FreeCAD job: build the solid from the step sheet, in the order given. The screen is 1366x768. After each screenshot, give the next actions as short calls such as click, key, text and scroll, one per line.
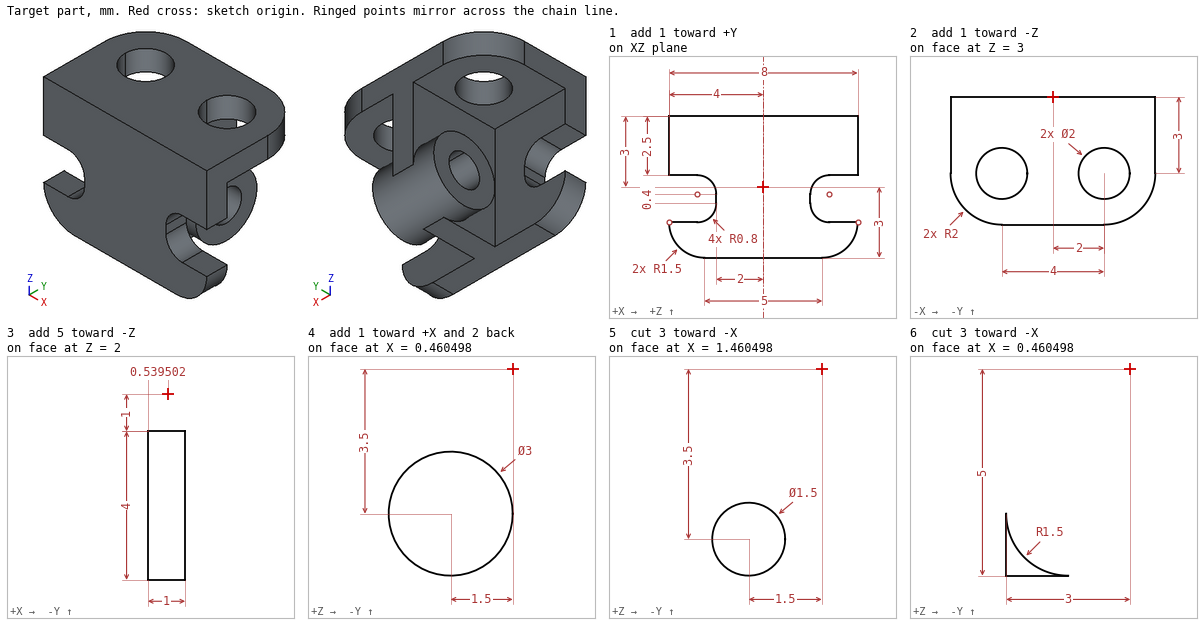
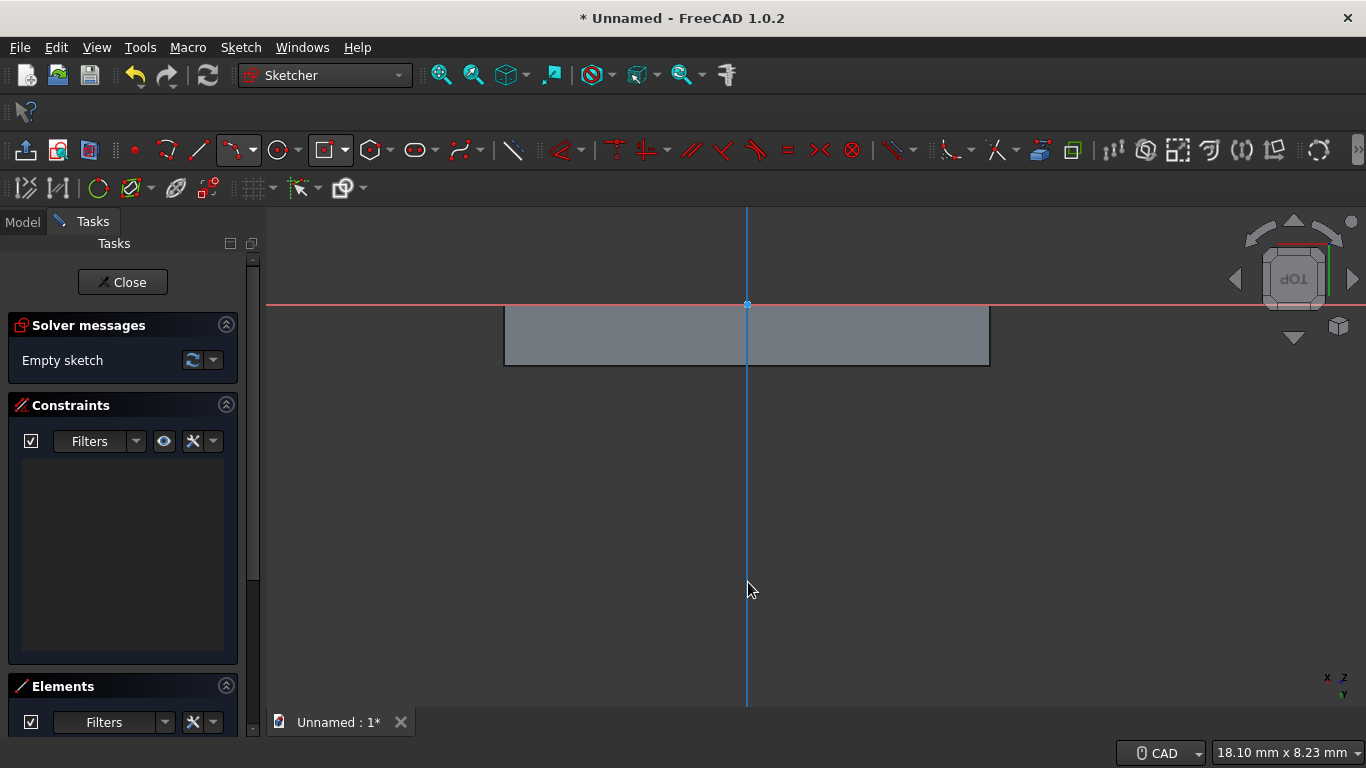
click(200, 150)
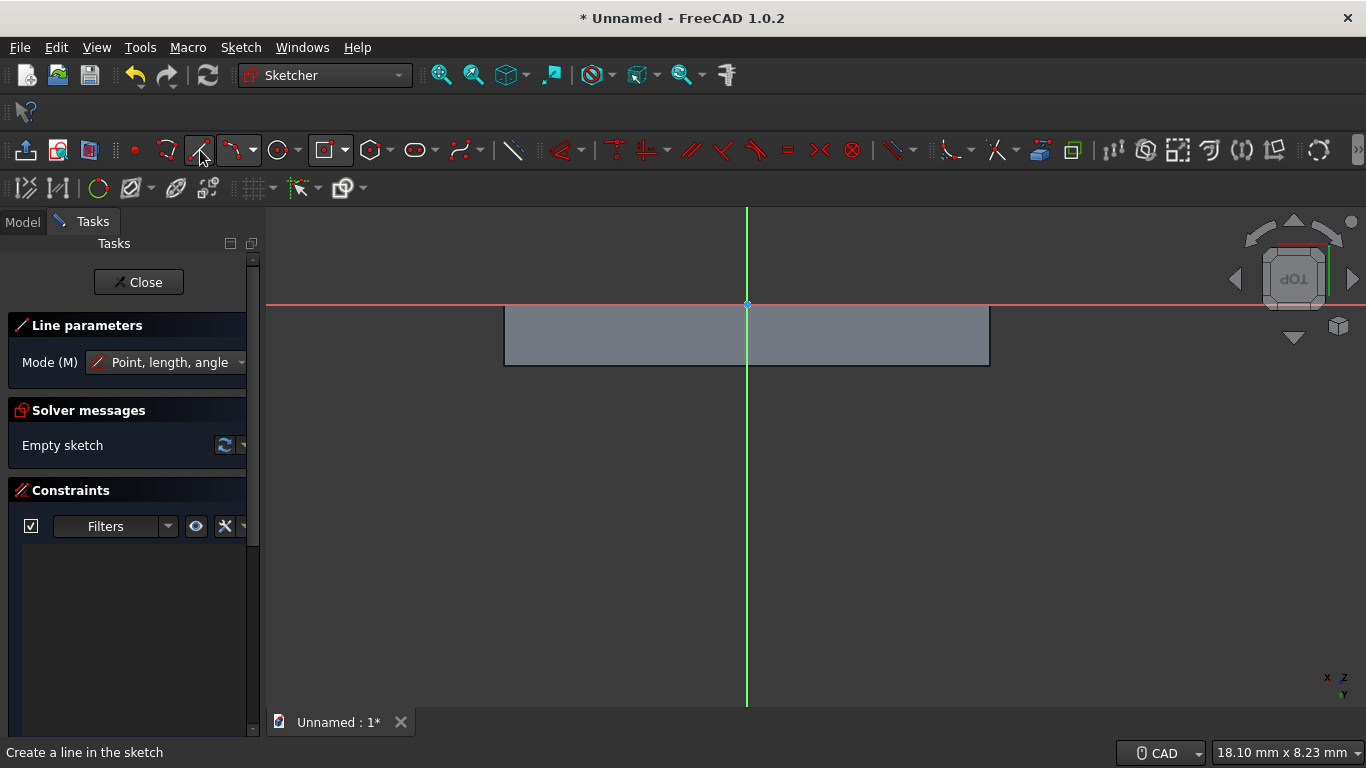
click(626, 609)
click(869, 609)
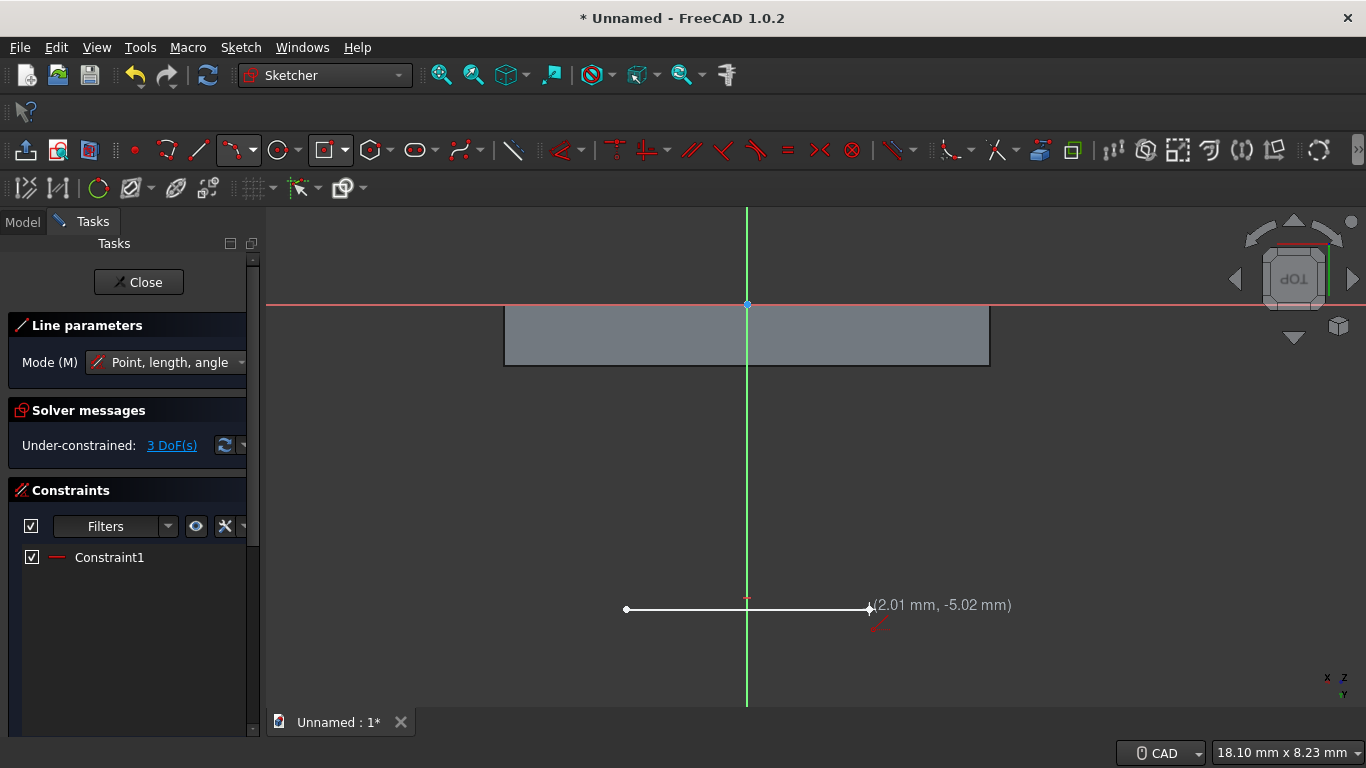
click(168, 150)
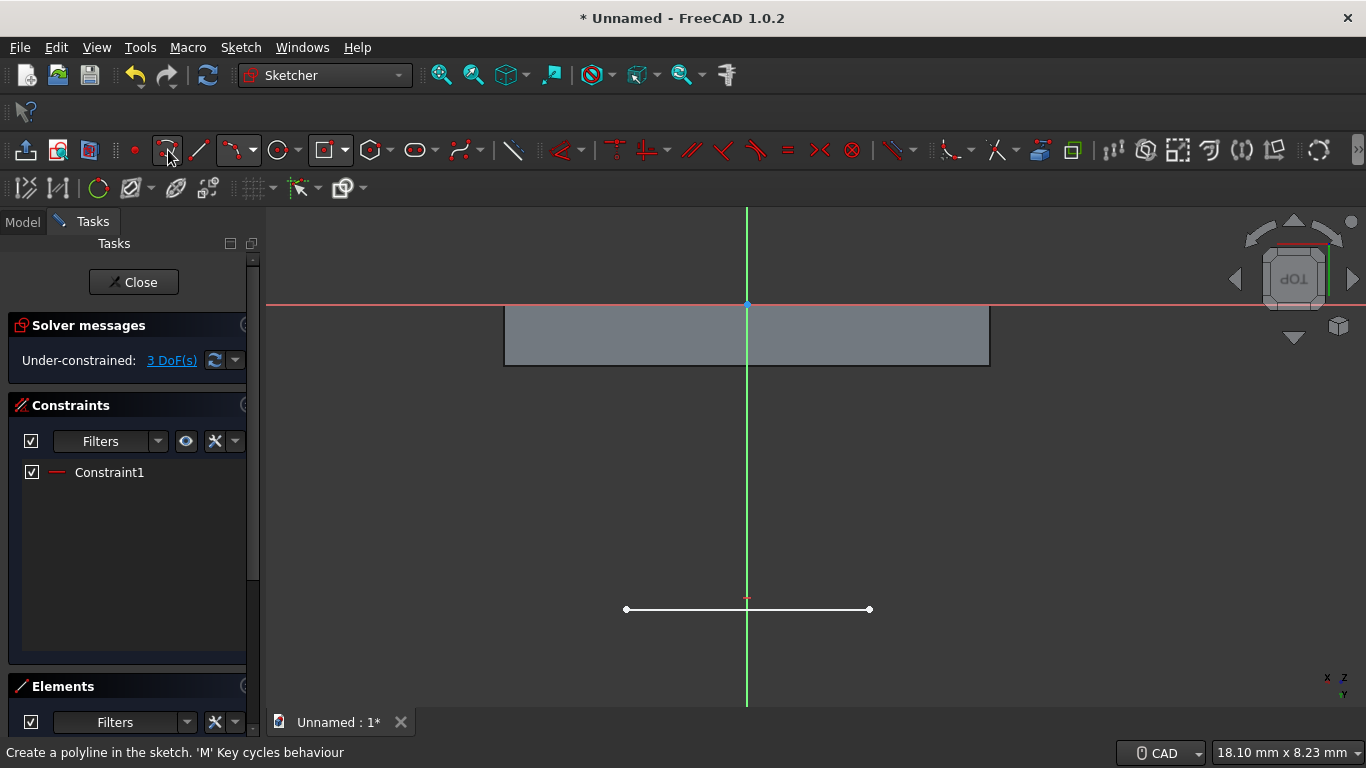
click(990, 487)
click(990, 305)
click(504, 314)
click(504, 487)
right_click(504, 487)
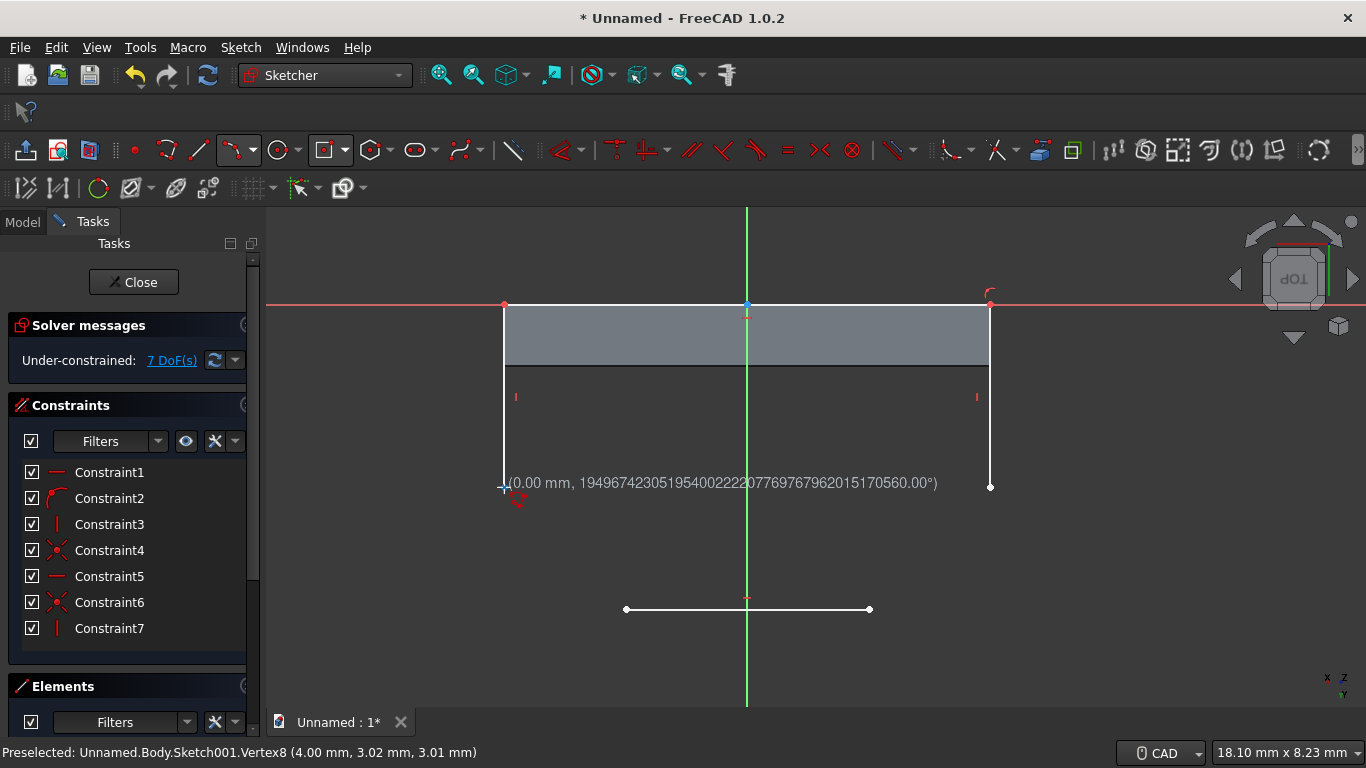
click(232, 150)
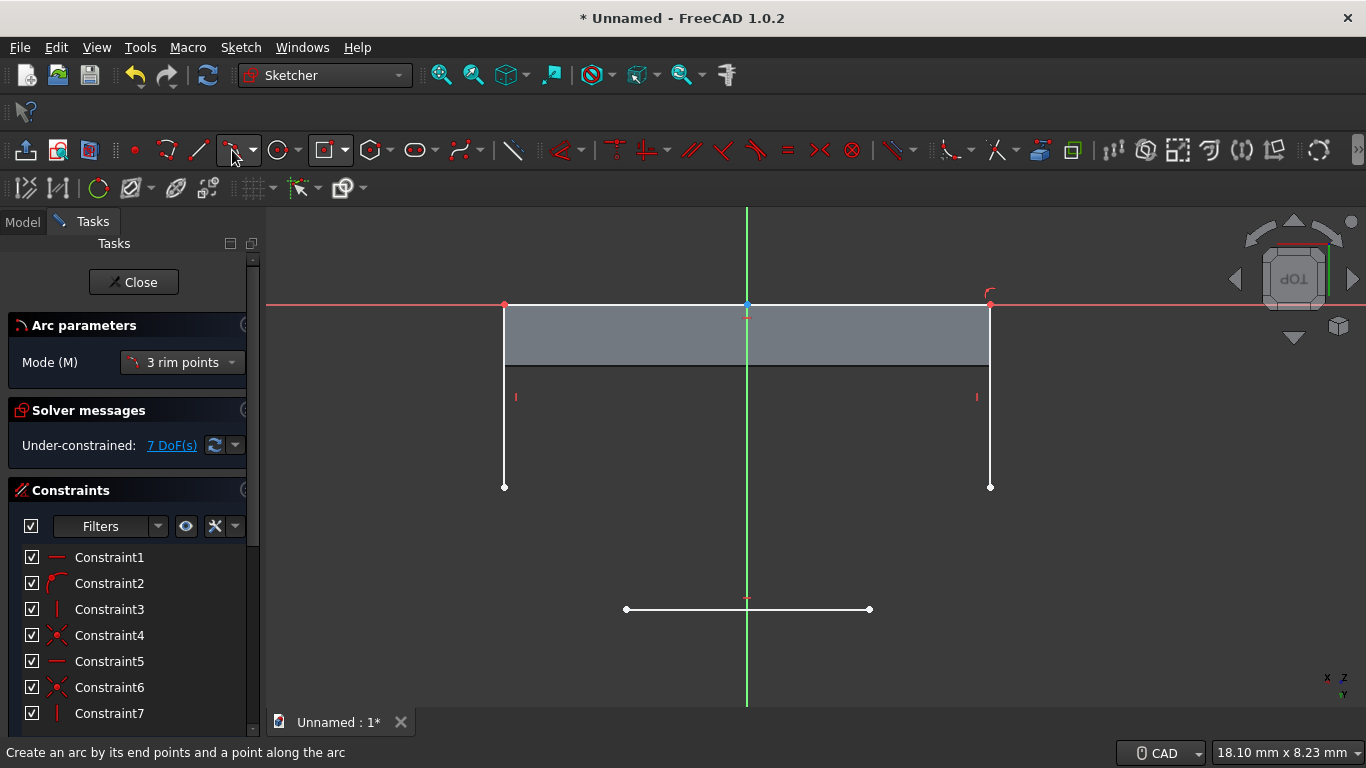
click(869, 610)
click(990, 488)
click(955, 573)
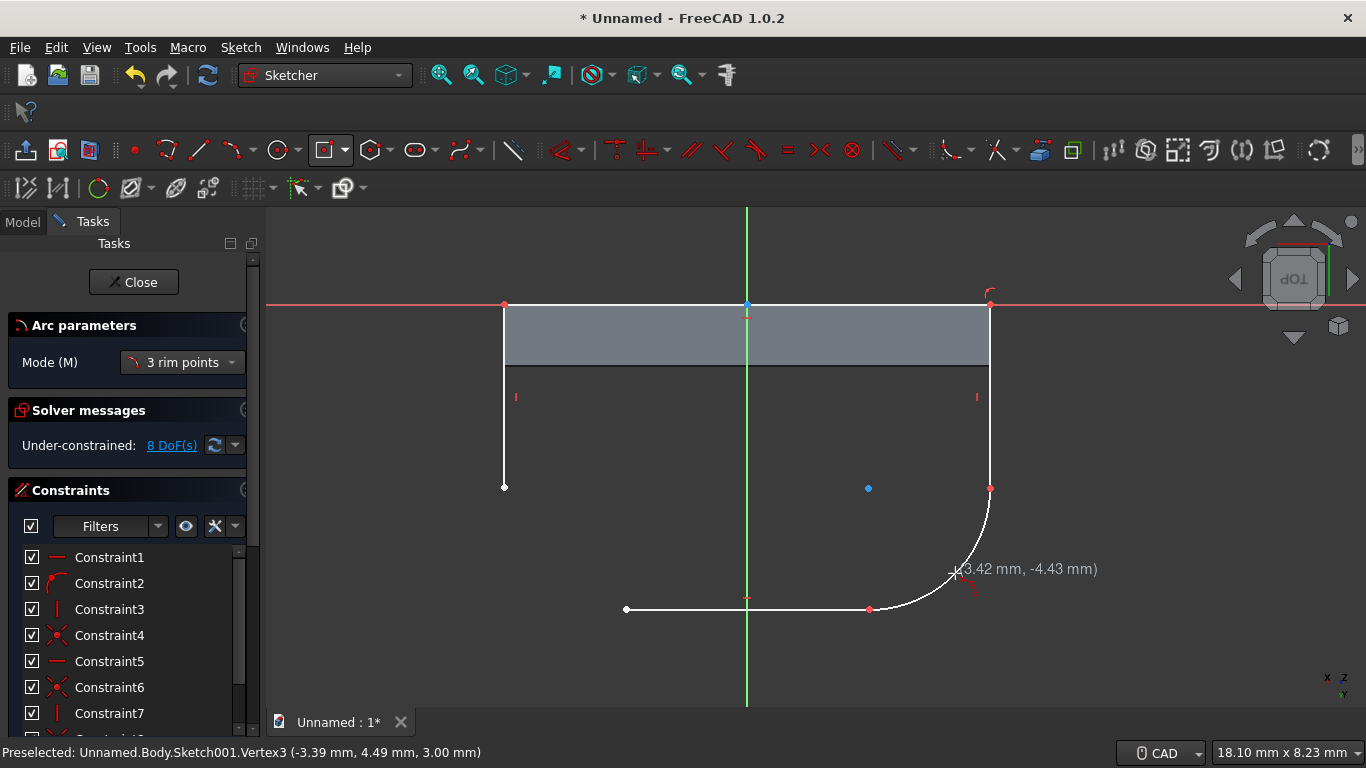
click(504, 488)
click(626, 610)
click(540, 573)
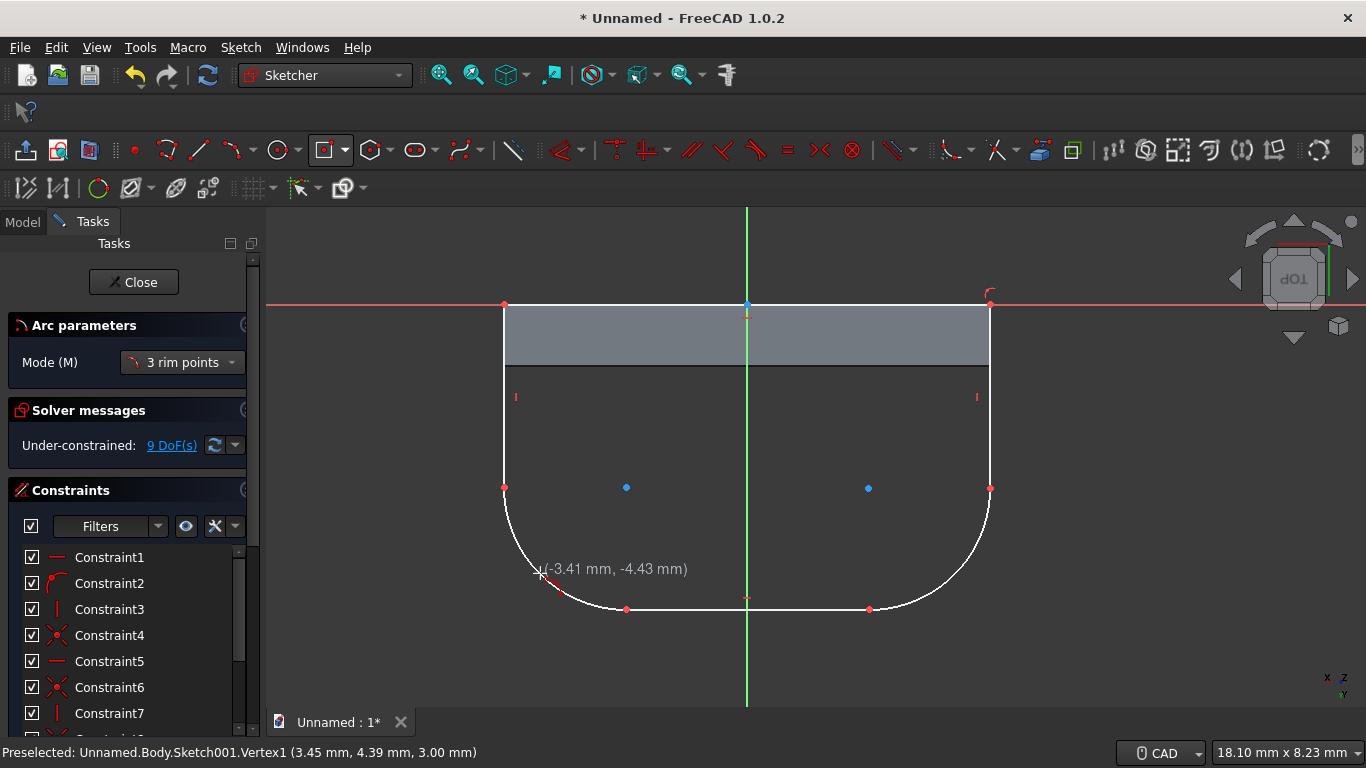
click(278, 150)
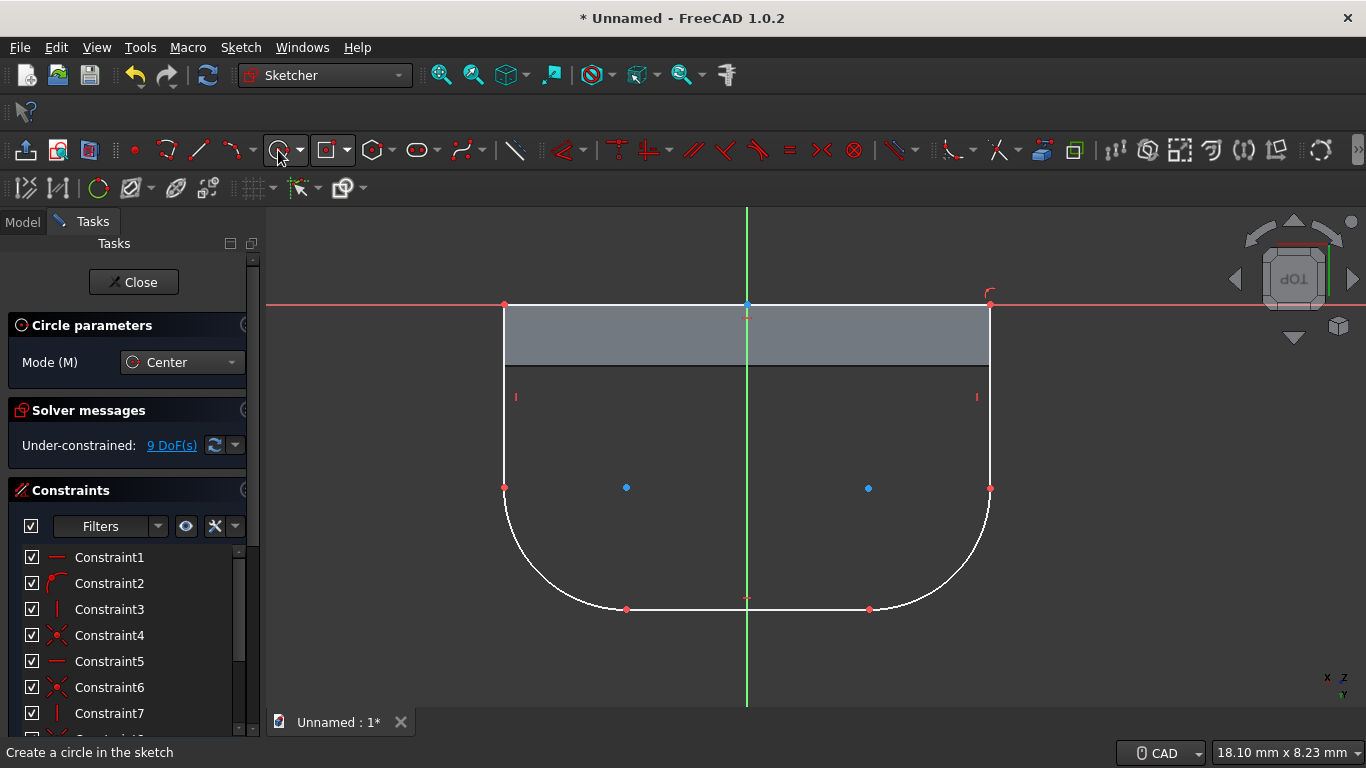
click(869, 487)
click(912, 444)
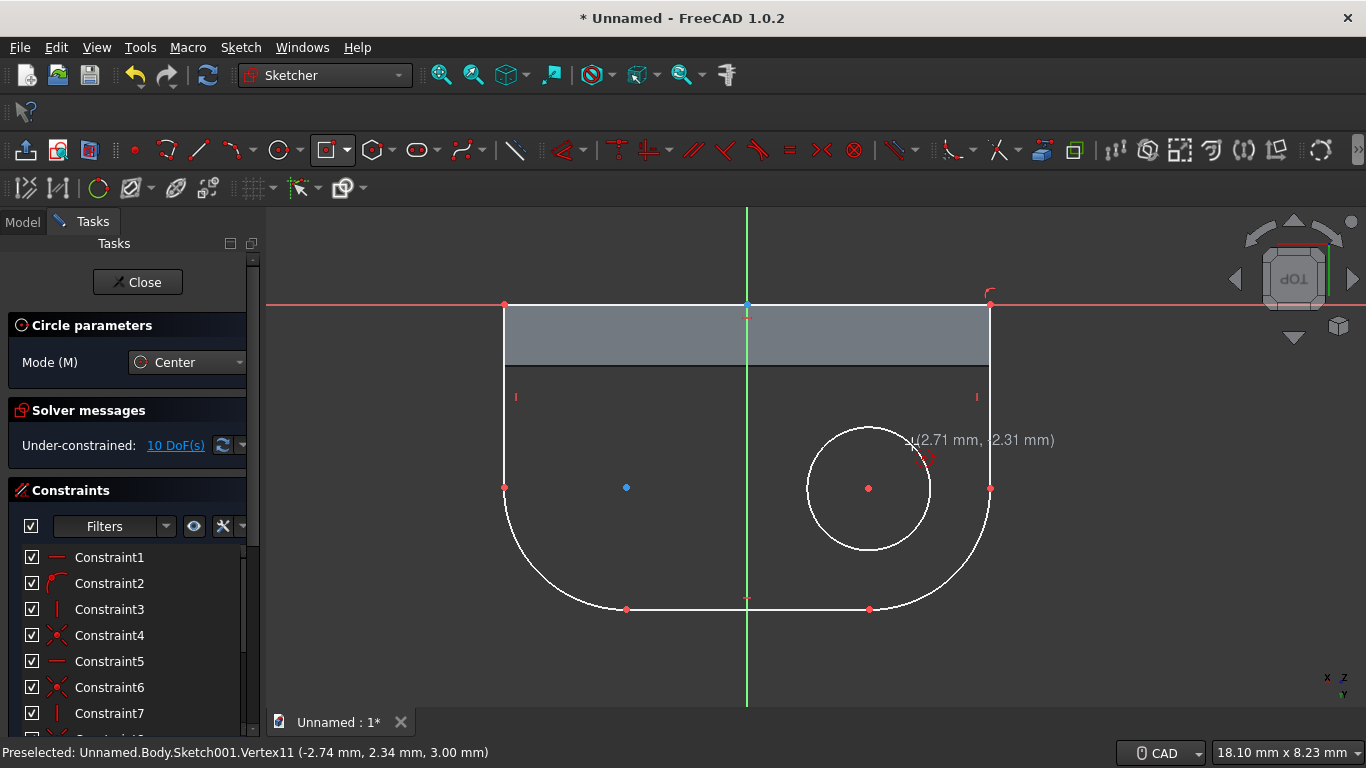
click(626, 487)
click(668, 444)
key(Escape)